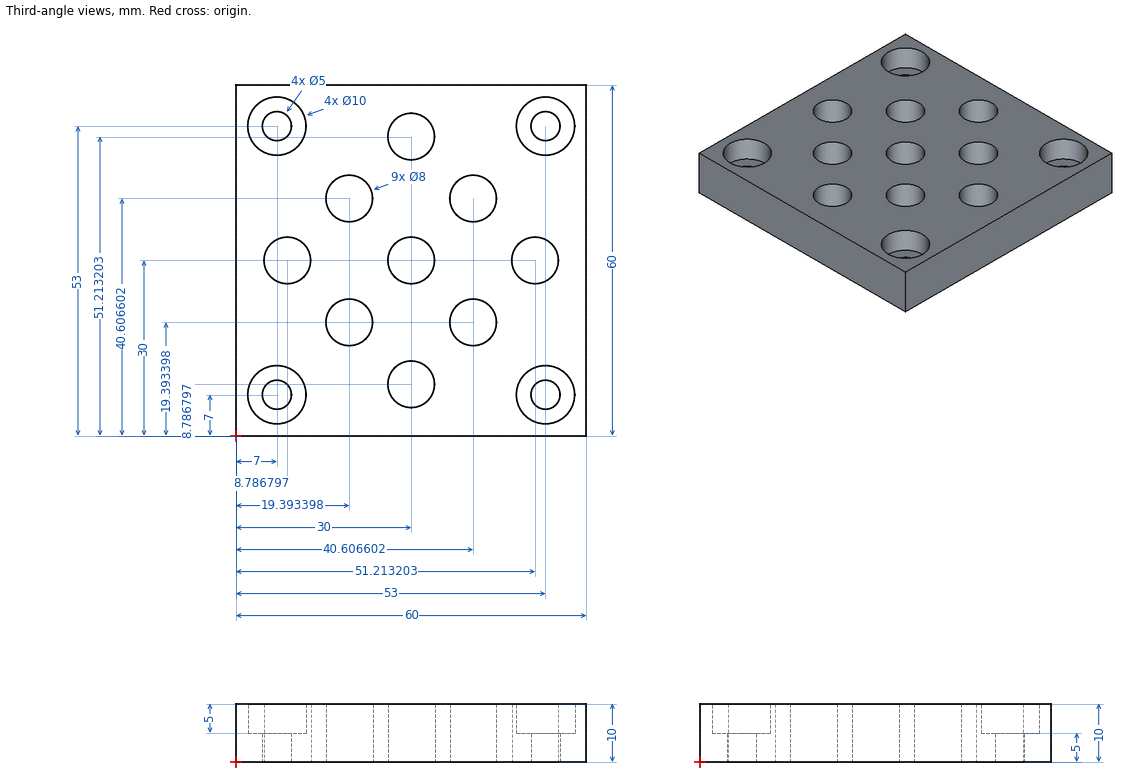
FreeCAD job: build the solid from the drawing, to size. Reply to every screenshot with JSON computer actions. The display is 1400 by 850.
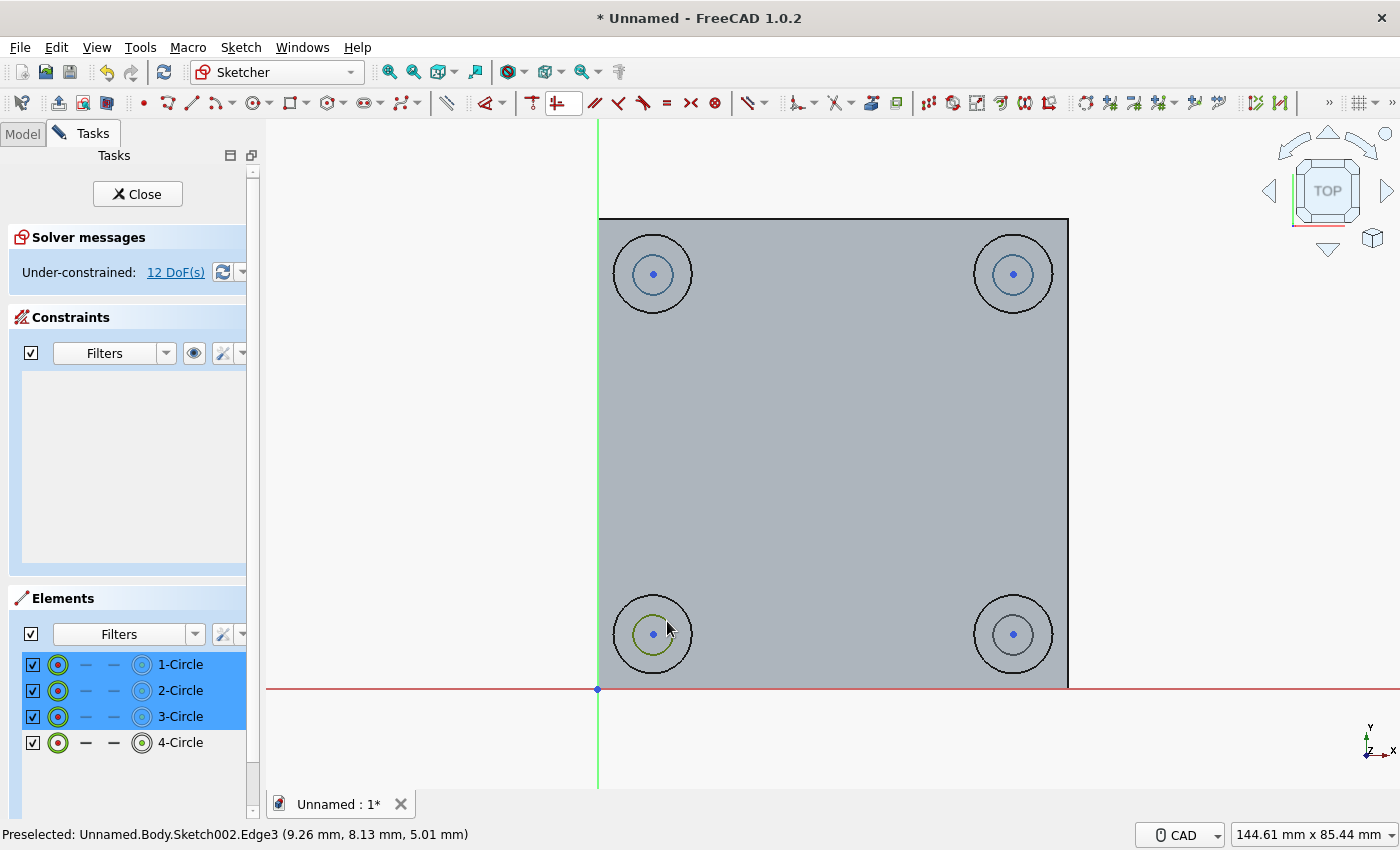
{"action": "left_click", "coordinate": [1027, 621]}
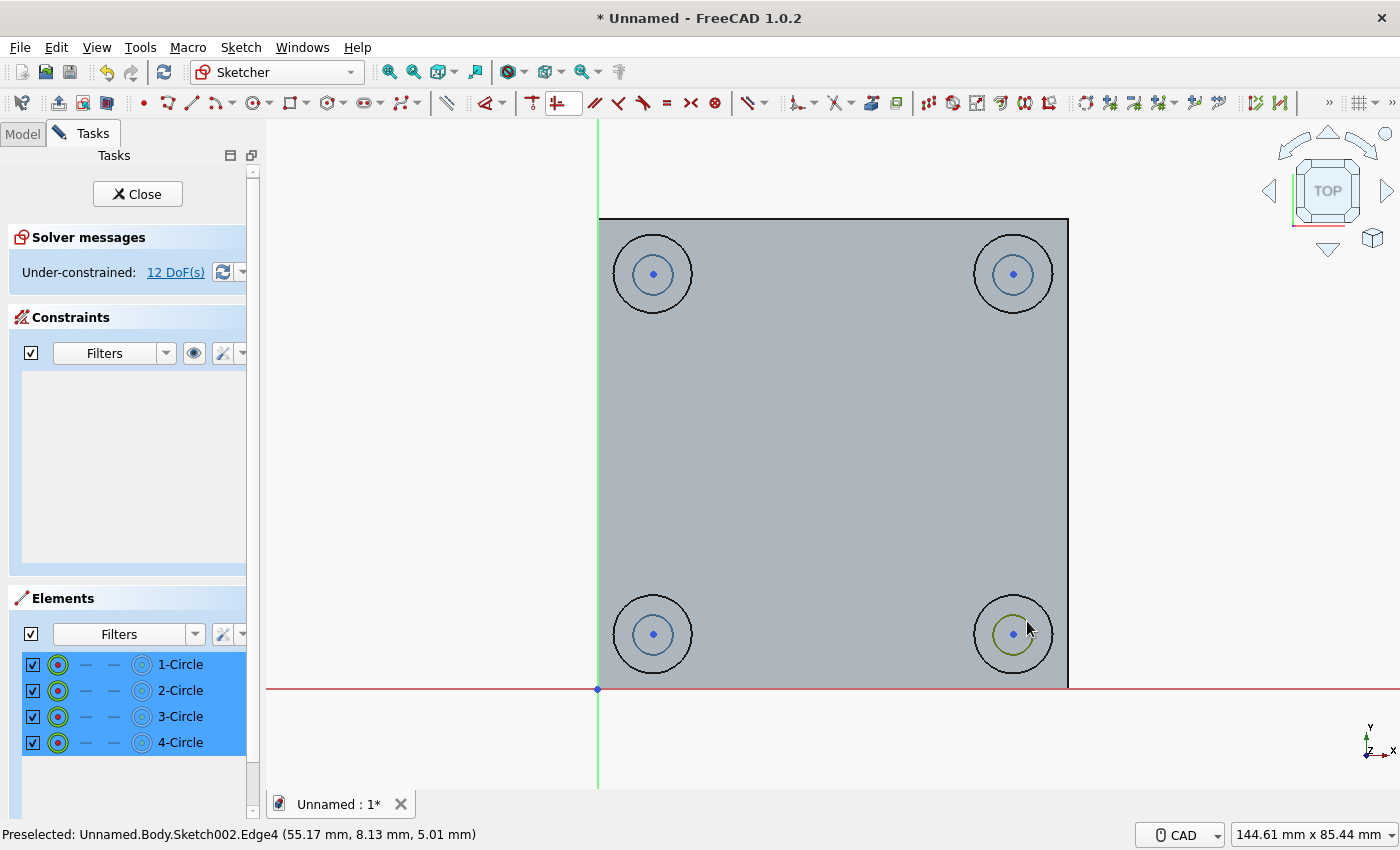
{"action": "key", "text": "e"}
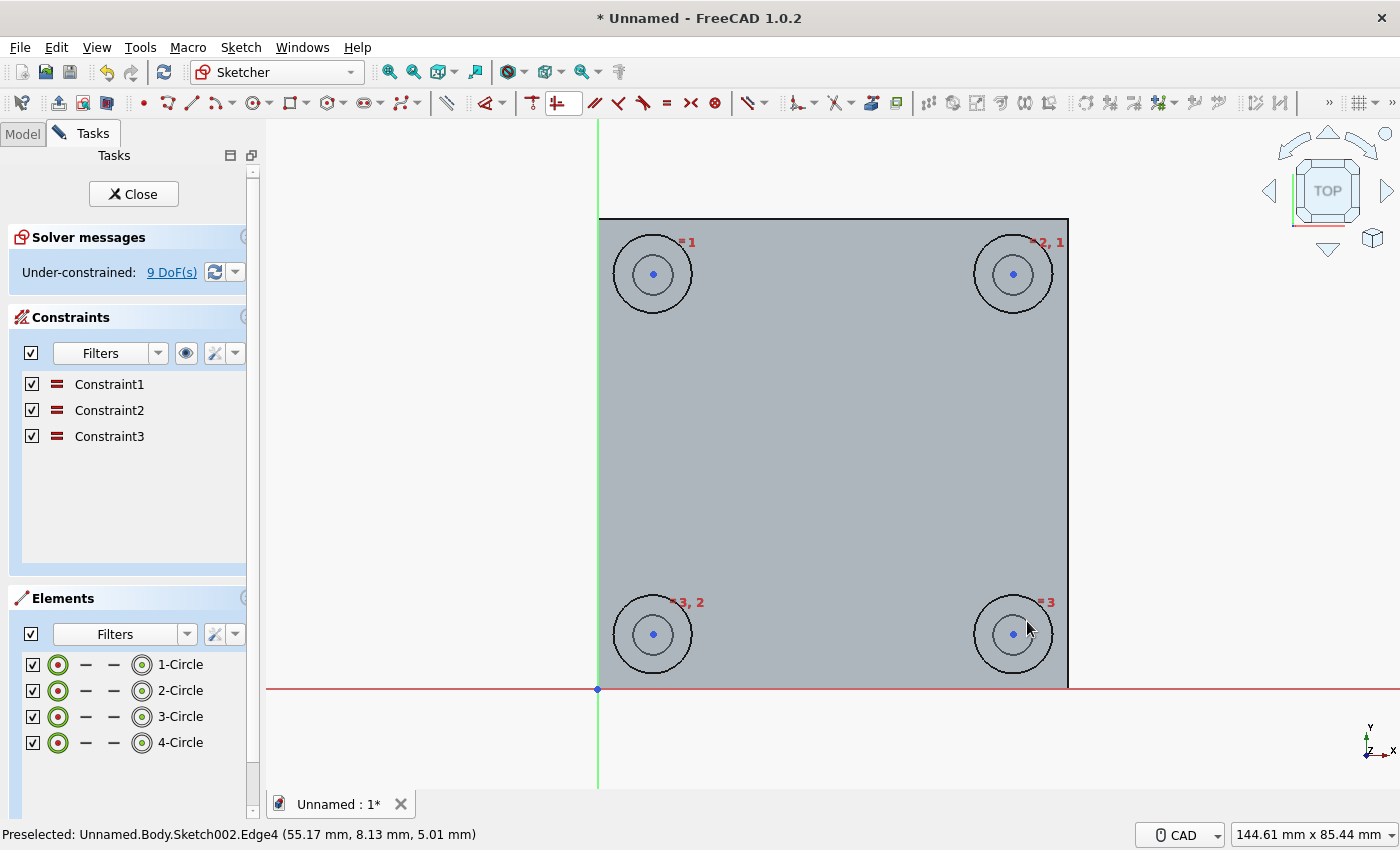
{"action": "left_click", "coordinate": [653, 275]}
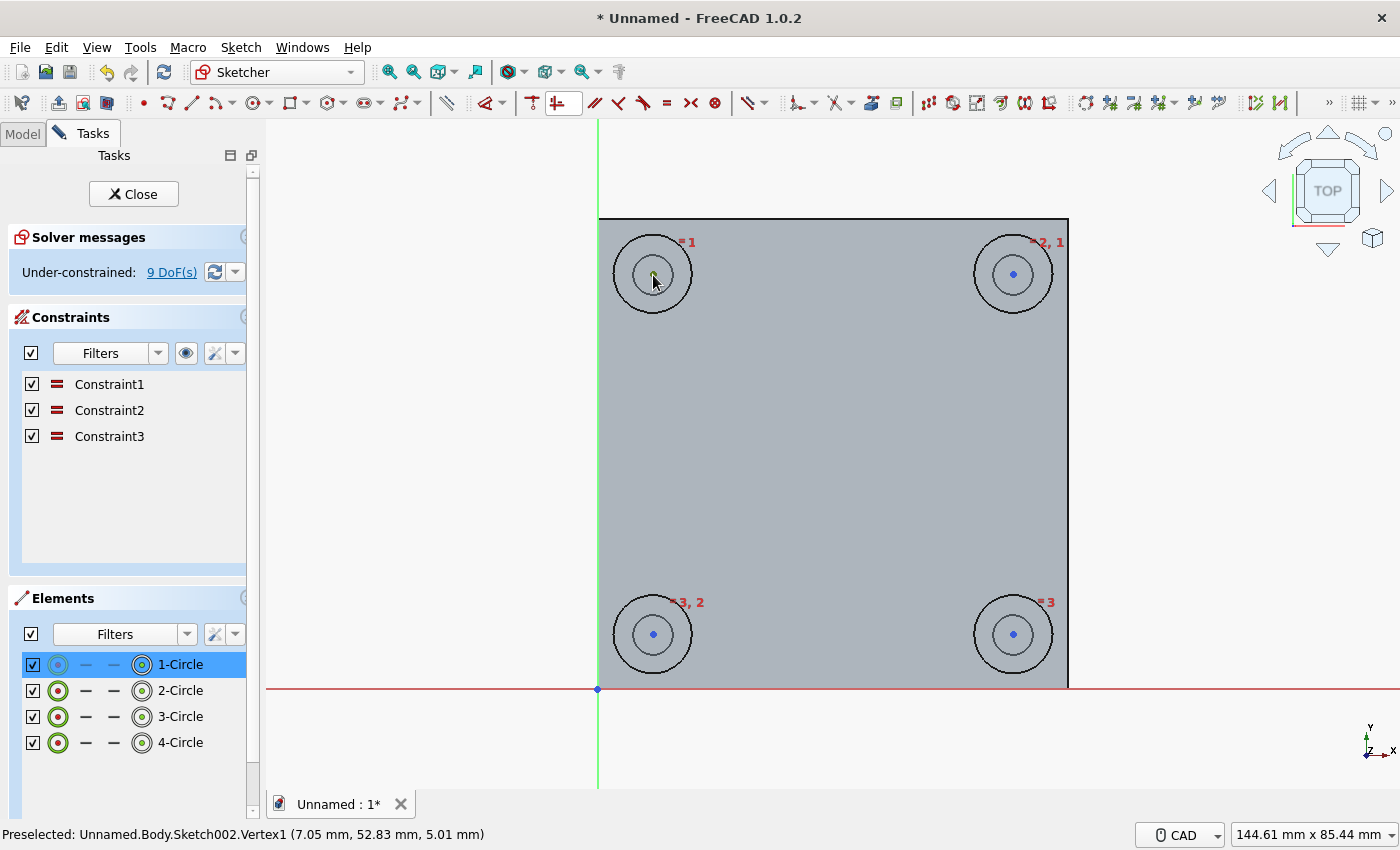
{"action": "left_click", "coordinate": [1013, 275]}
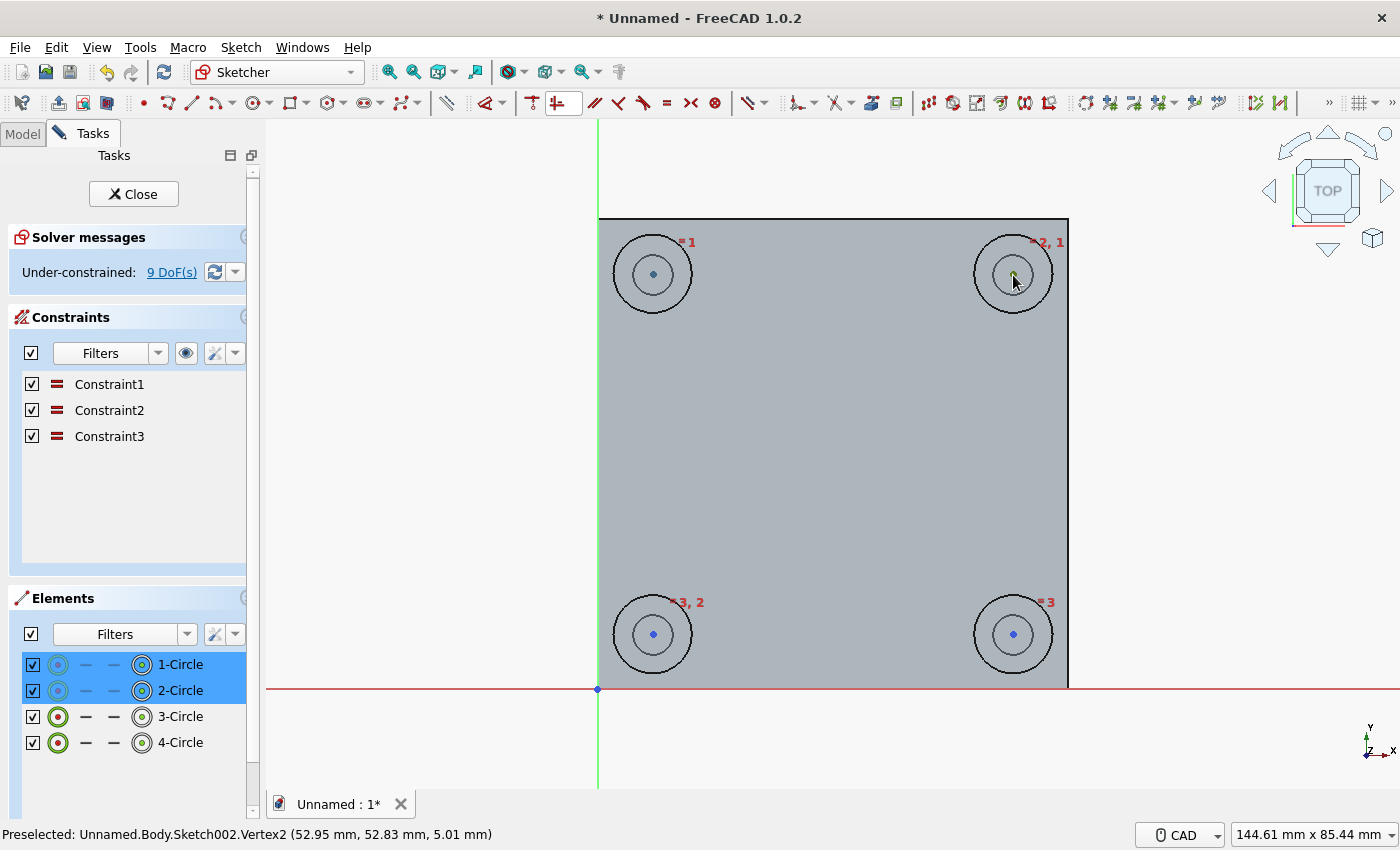
{"action": "left_click", "coordinate": [576, 104]}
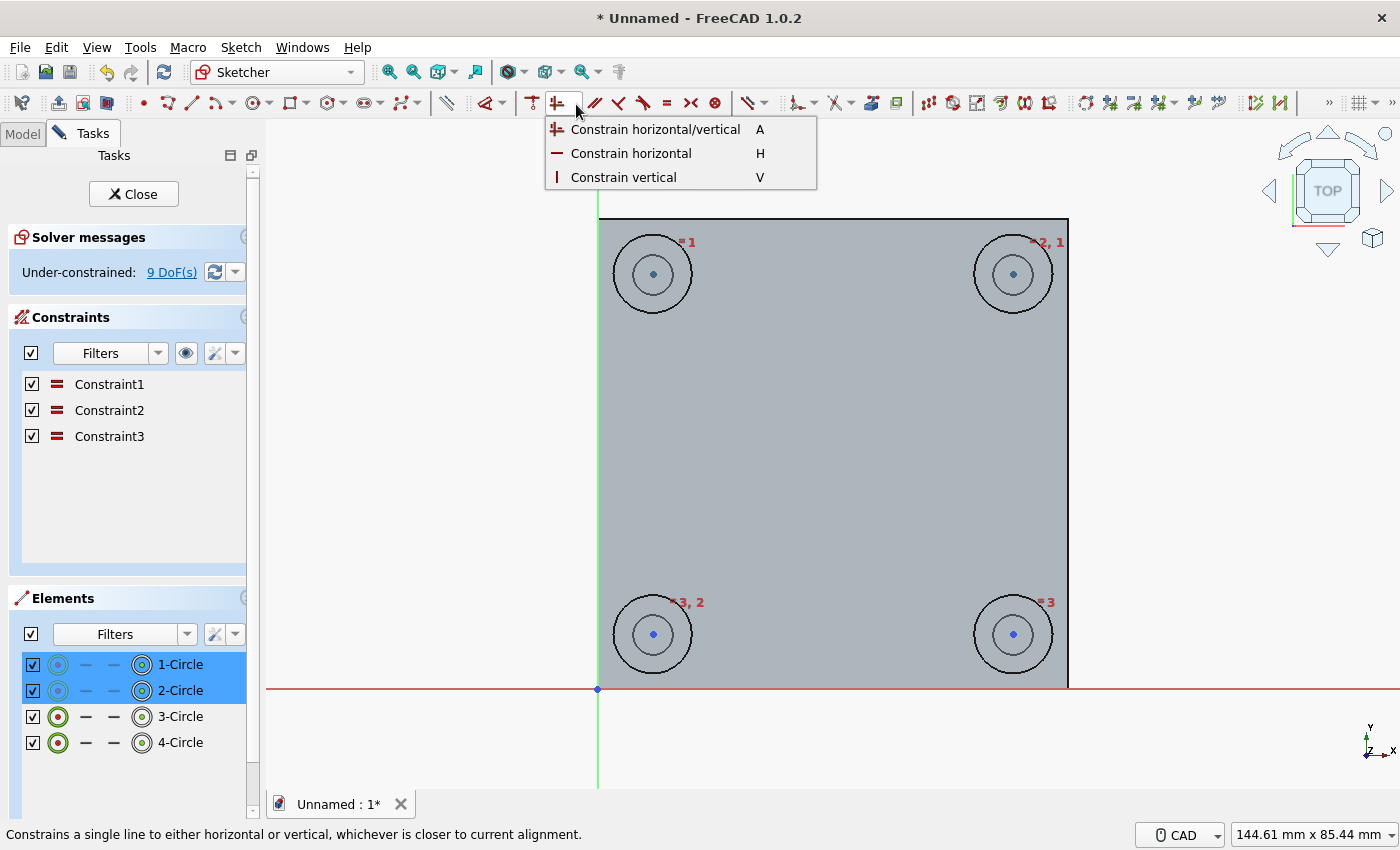
{"action": "left_click", "coordinate": [681, 153]}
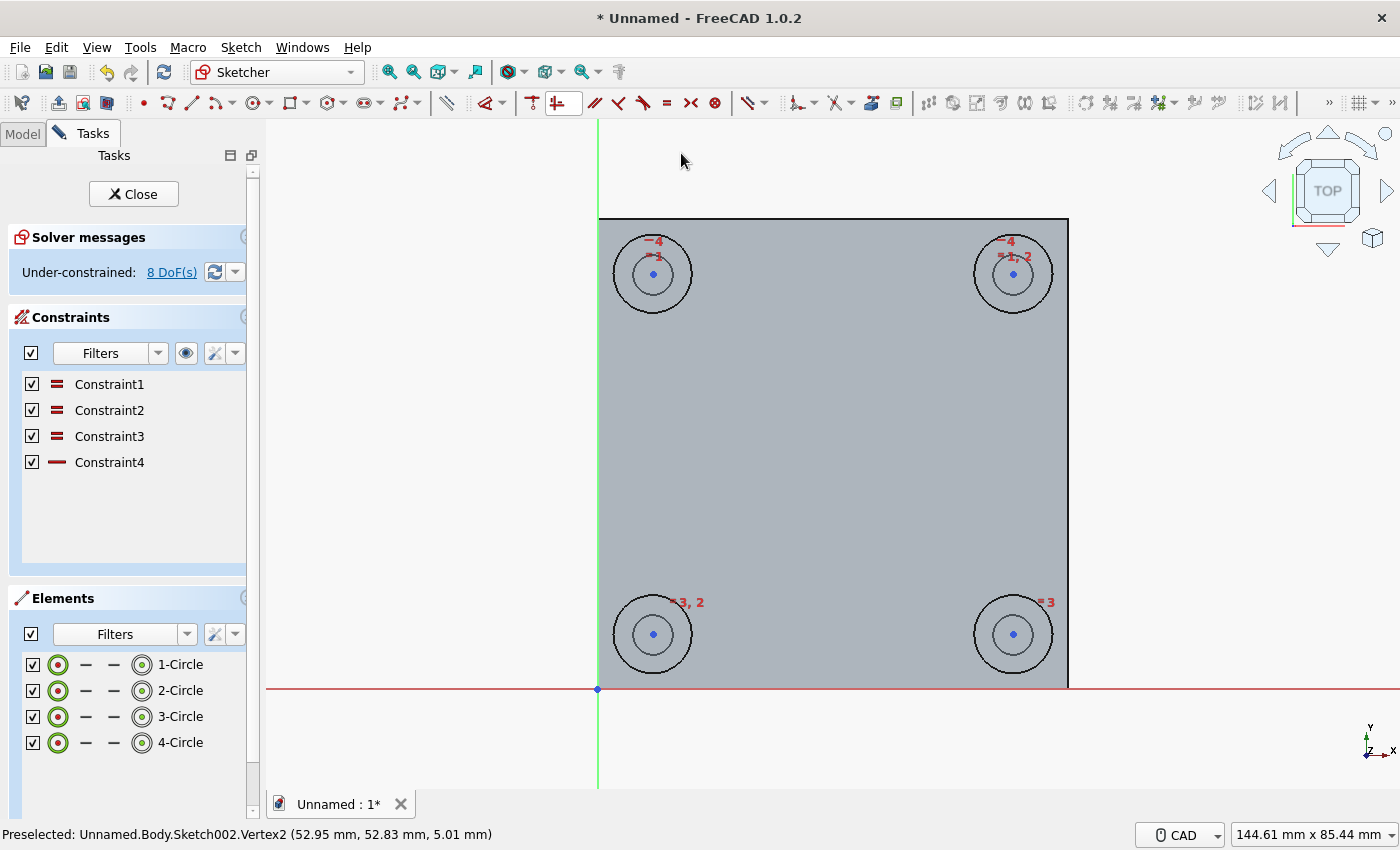
{"action": "left_click", "coordinate": [653, 275]}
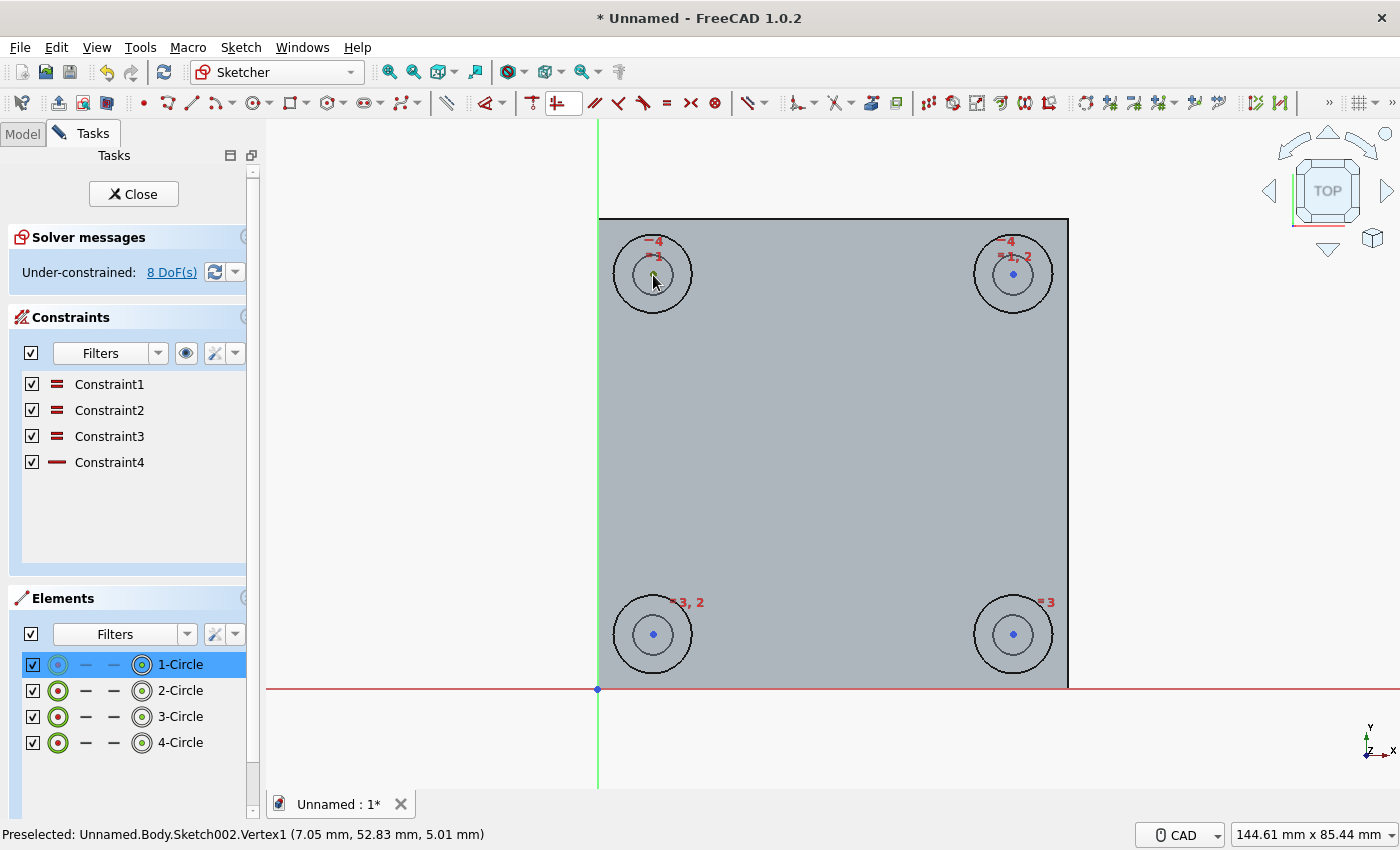
{"action": "left_click", "coordinate": [653, 635]}